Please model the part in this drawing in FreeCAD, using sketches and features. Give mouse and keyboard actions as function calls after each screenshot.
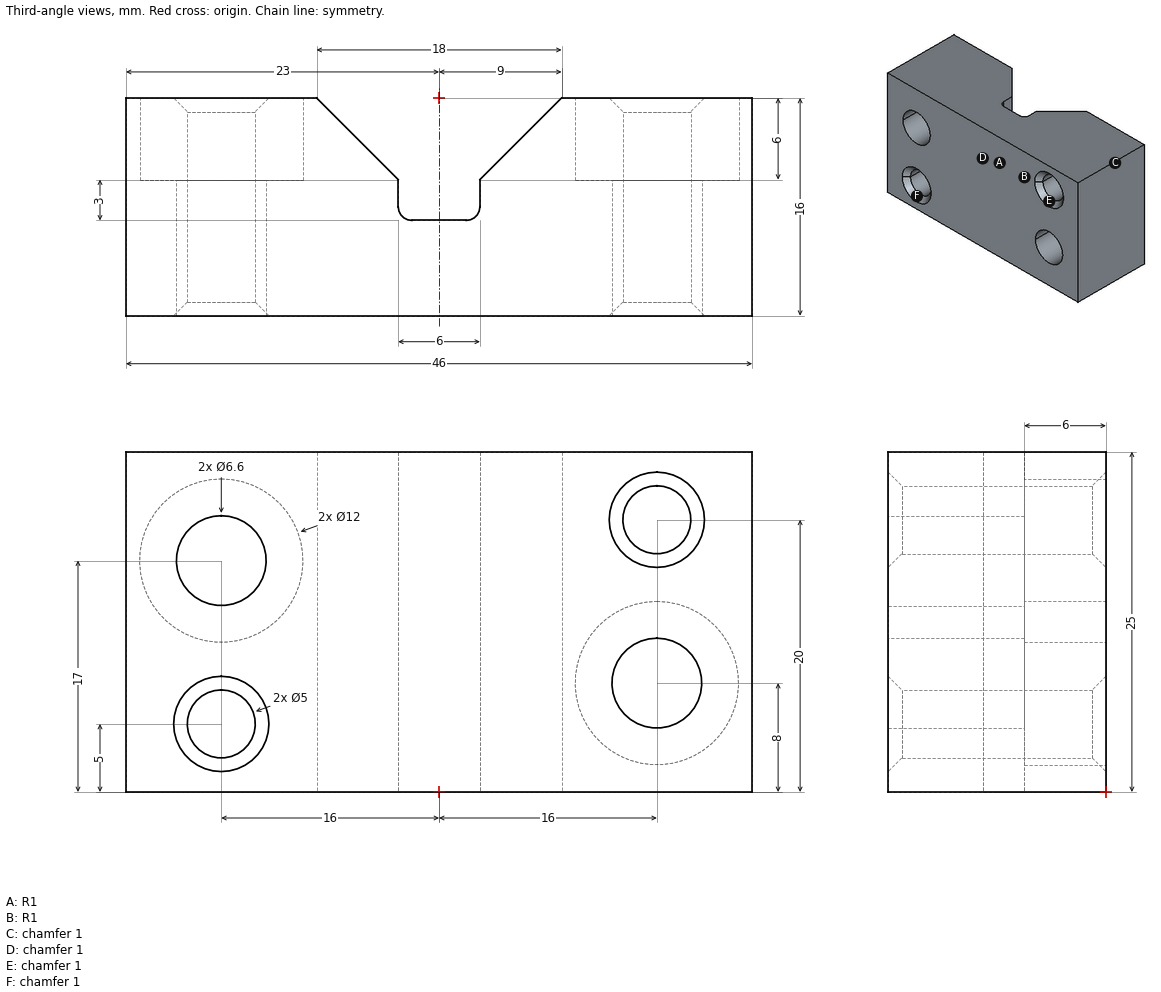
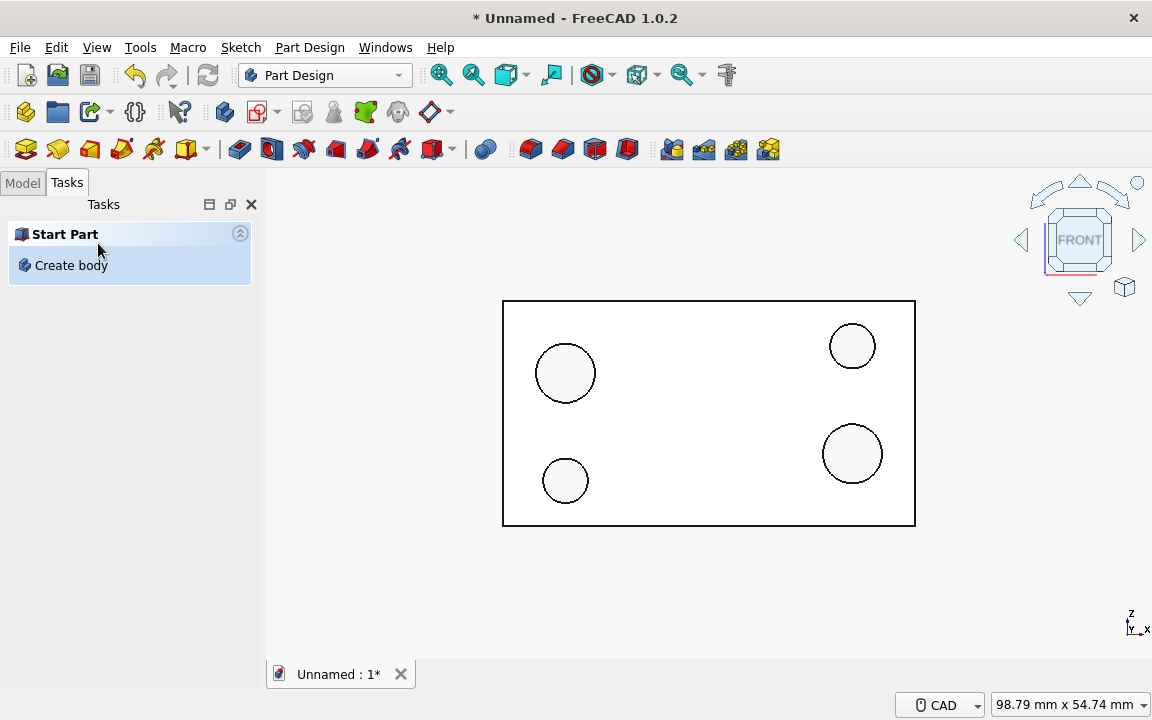
key(3)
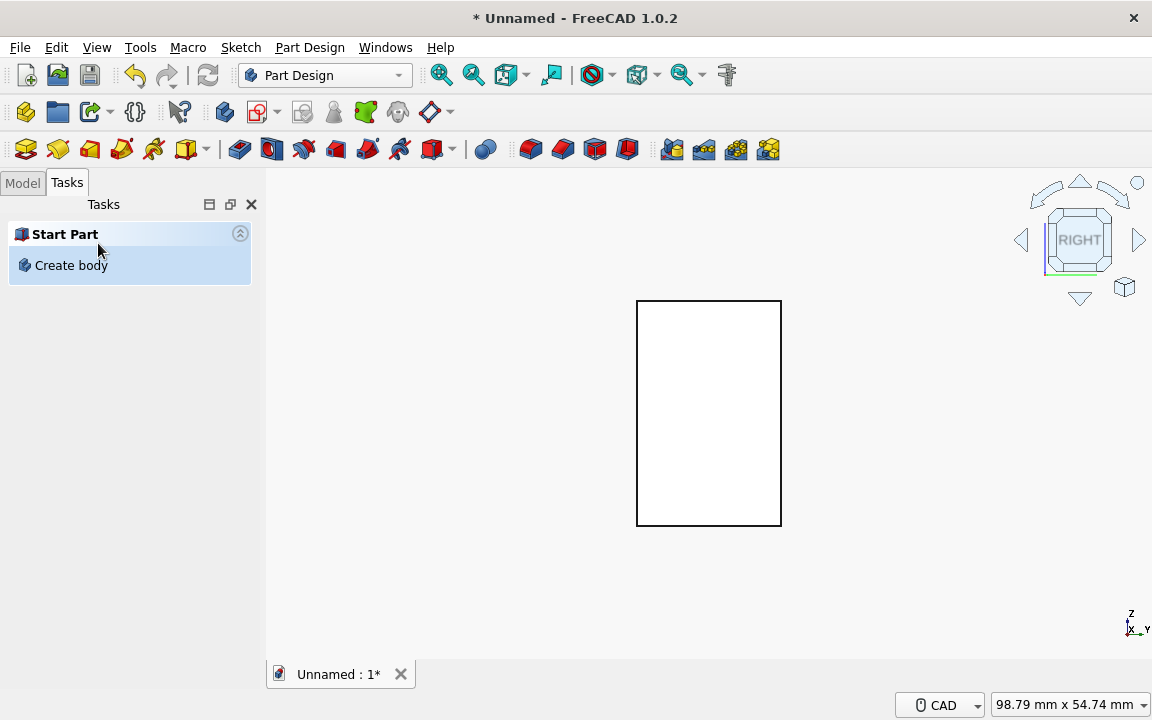
key(5)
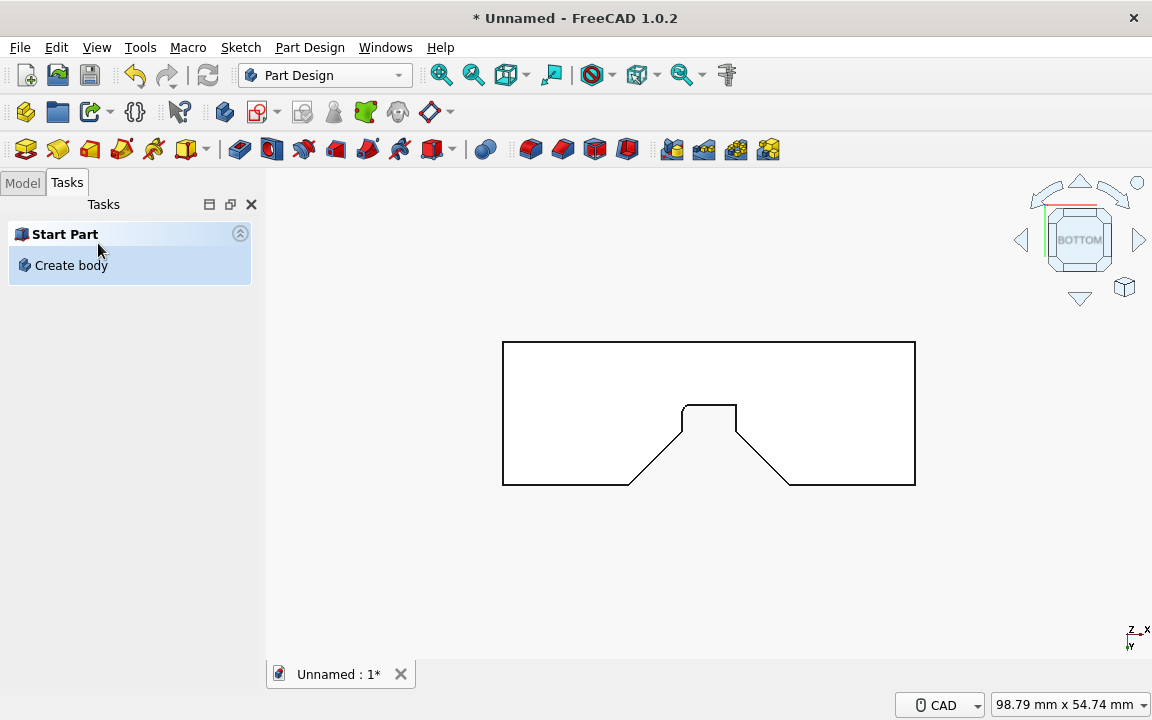
key(4)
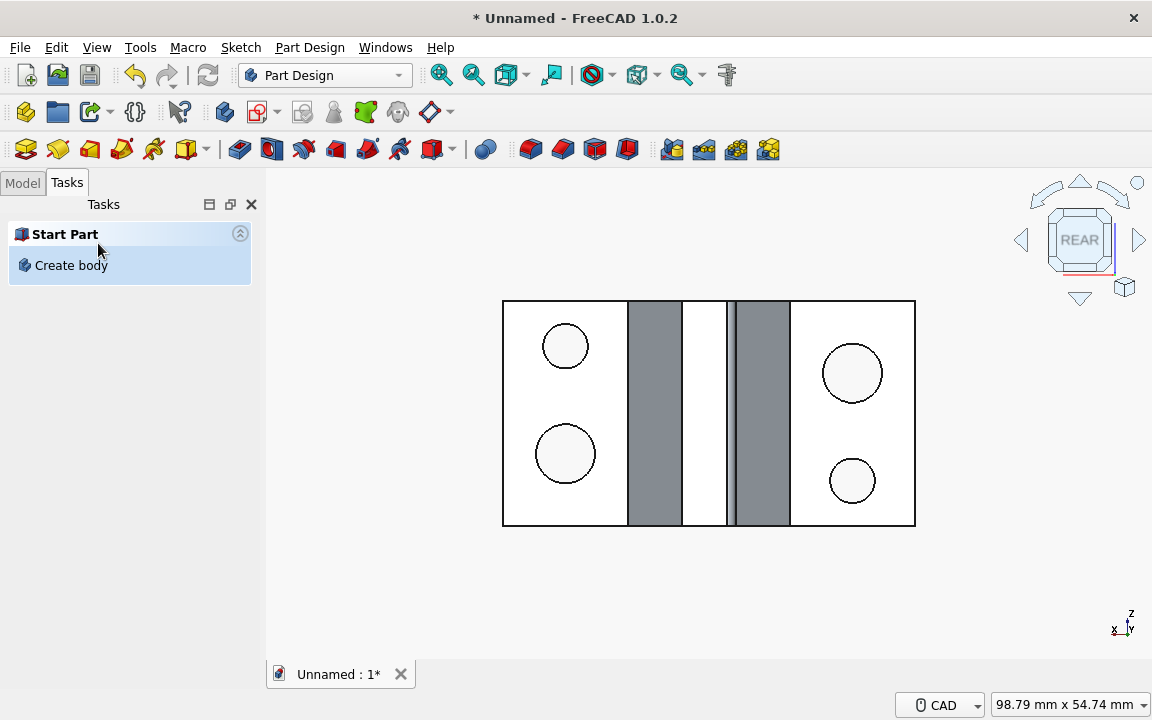
key(6)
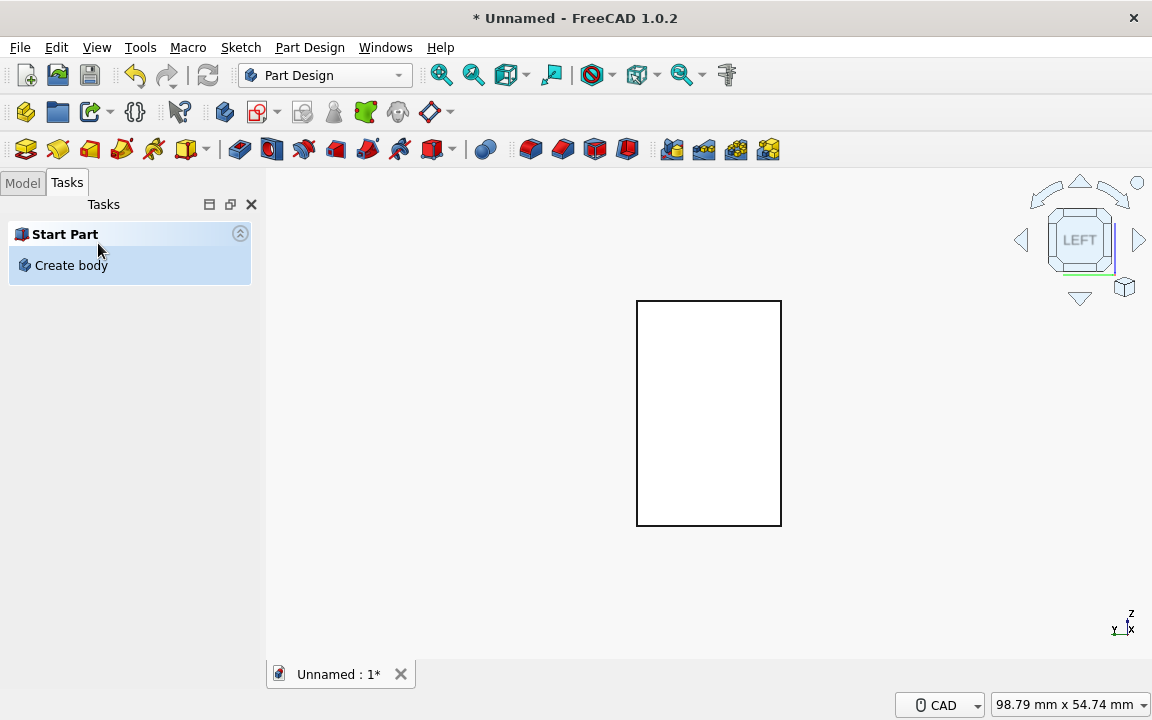
key(v)
key(3)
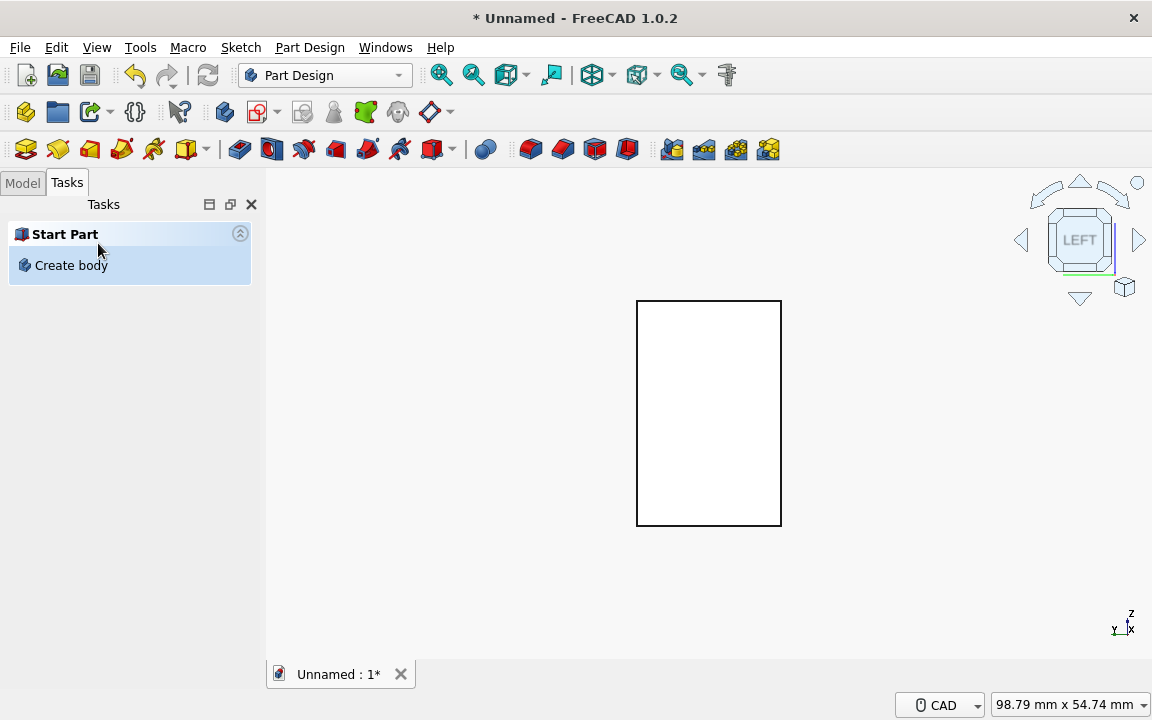
key(0)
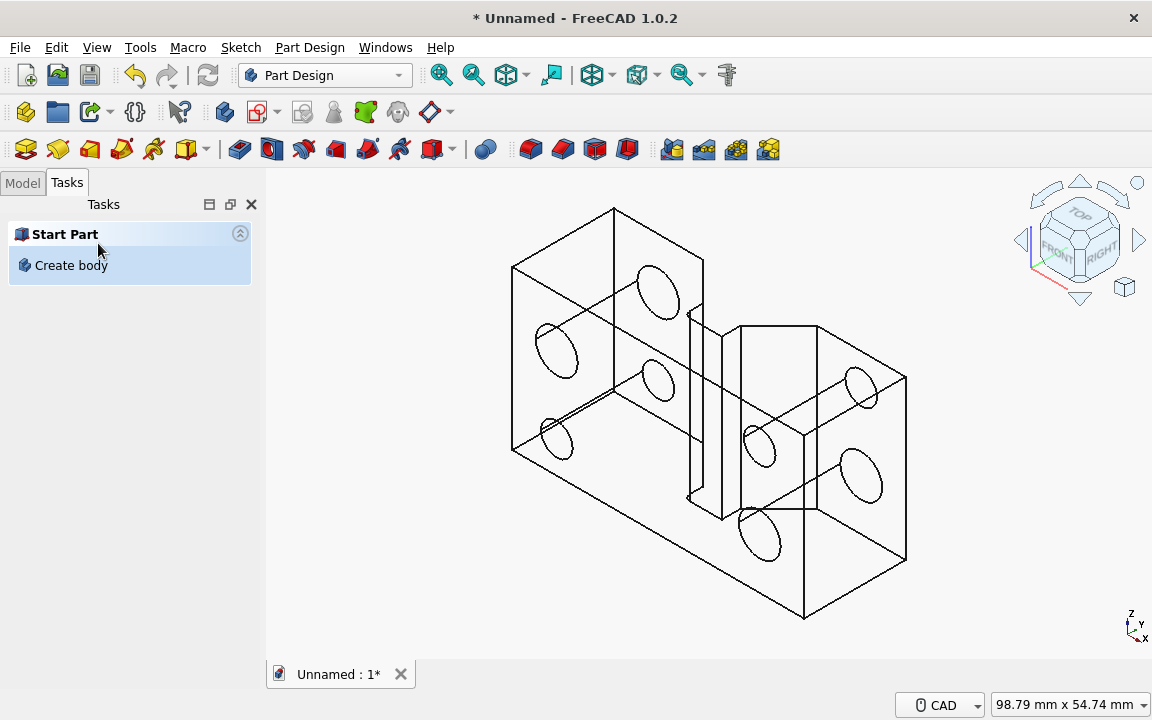
click(722, 427)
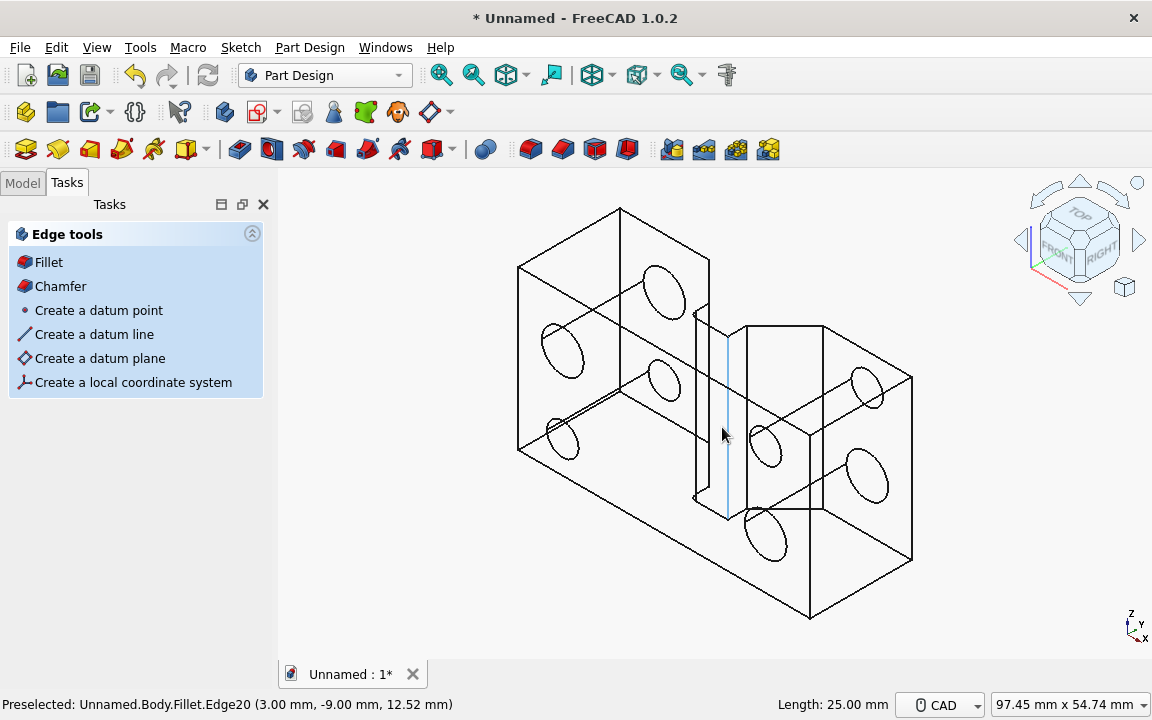
key(v)
key(1)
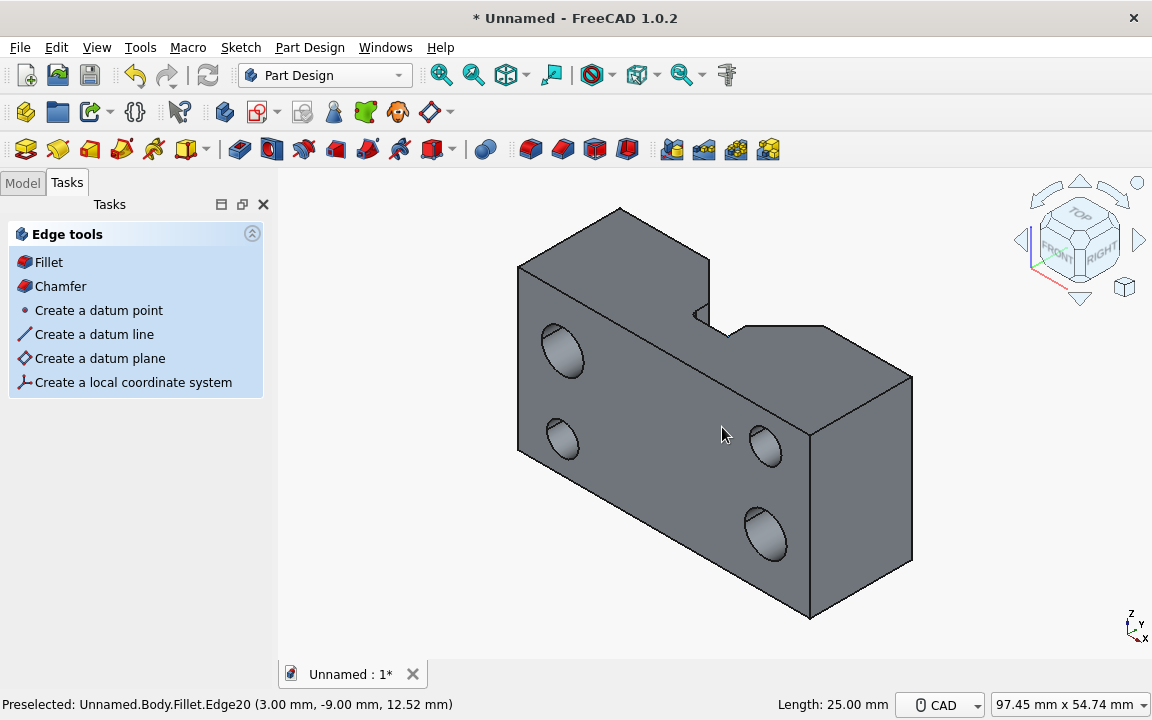
click(532, 150)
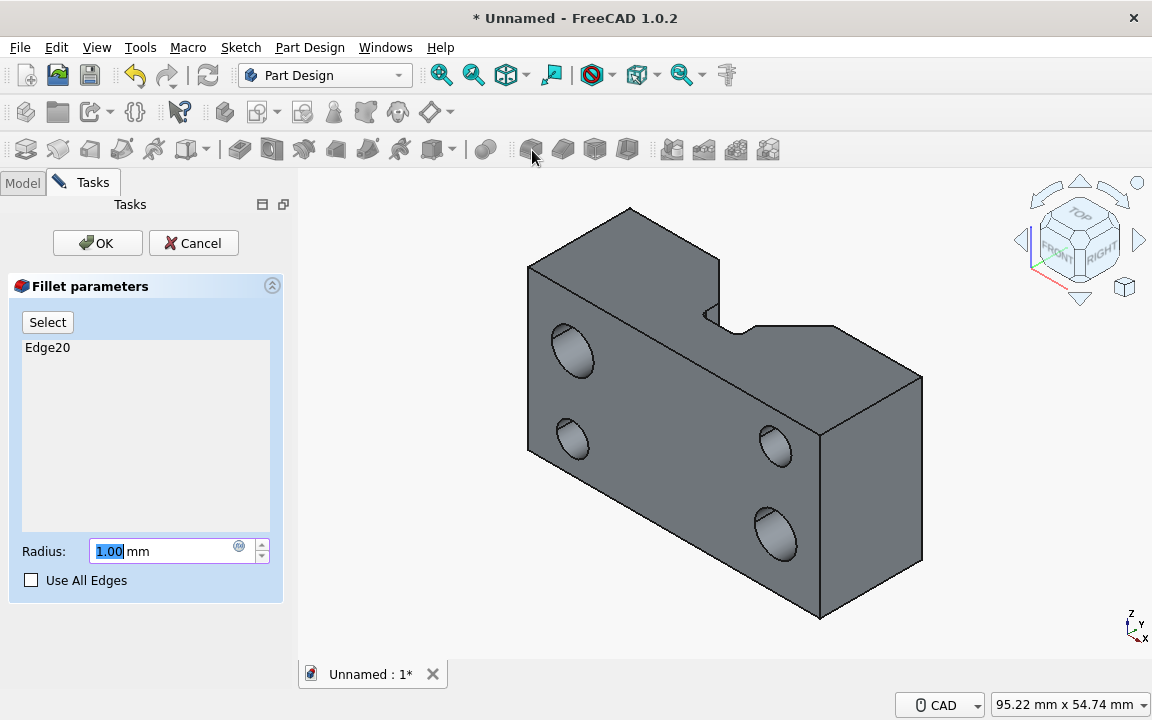
text(1)
key(Tab)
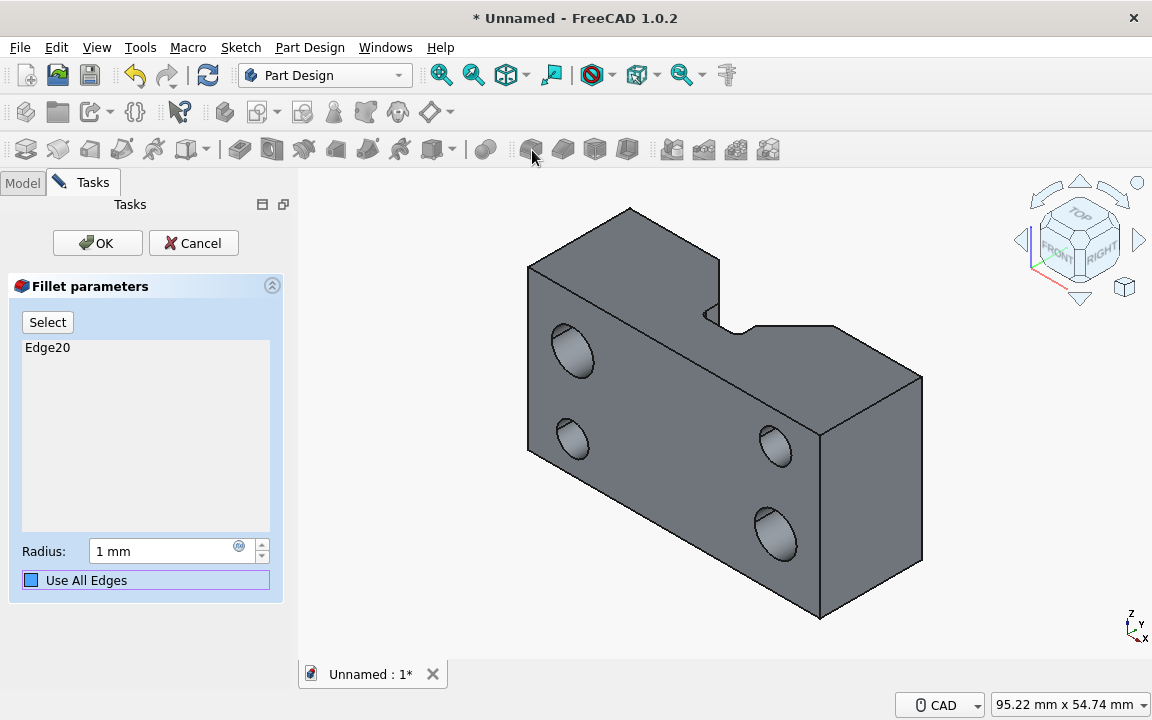
click(98, 243)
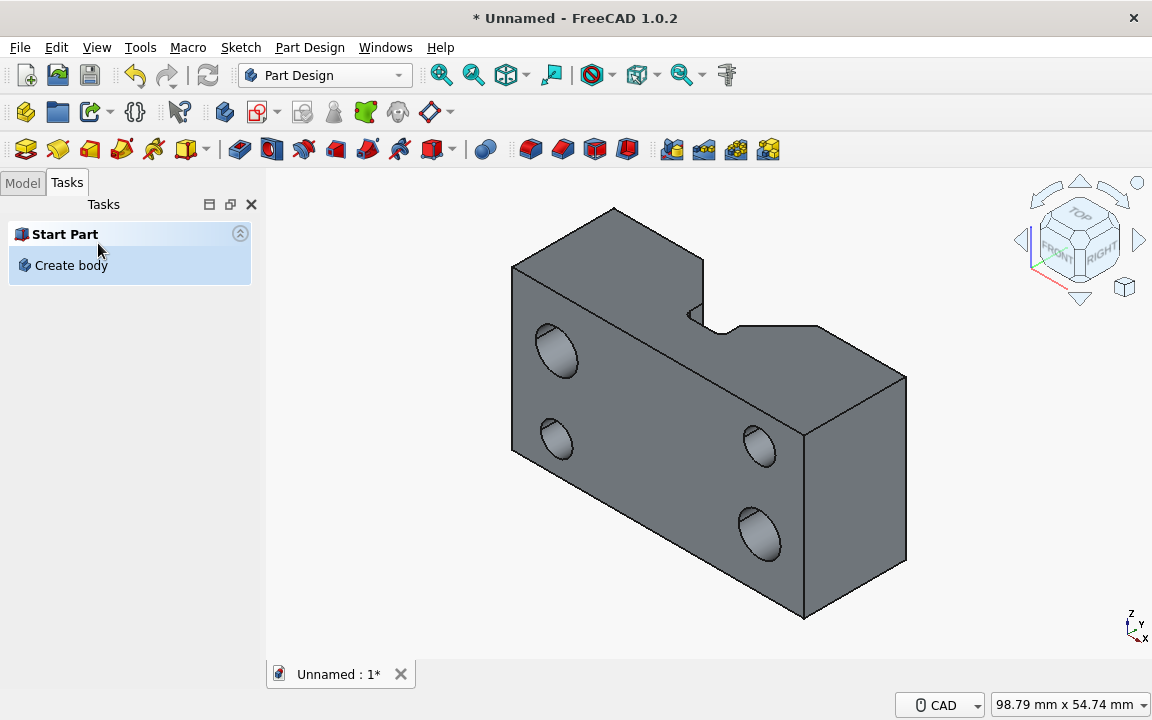
key(4)